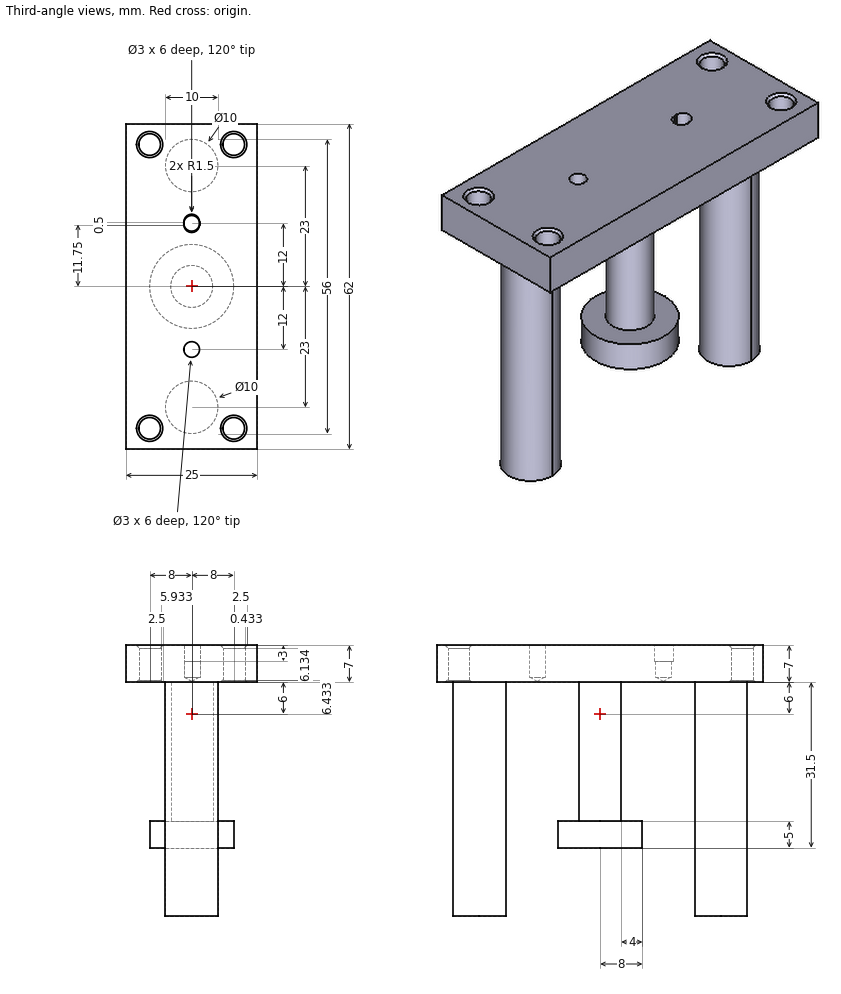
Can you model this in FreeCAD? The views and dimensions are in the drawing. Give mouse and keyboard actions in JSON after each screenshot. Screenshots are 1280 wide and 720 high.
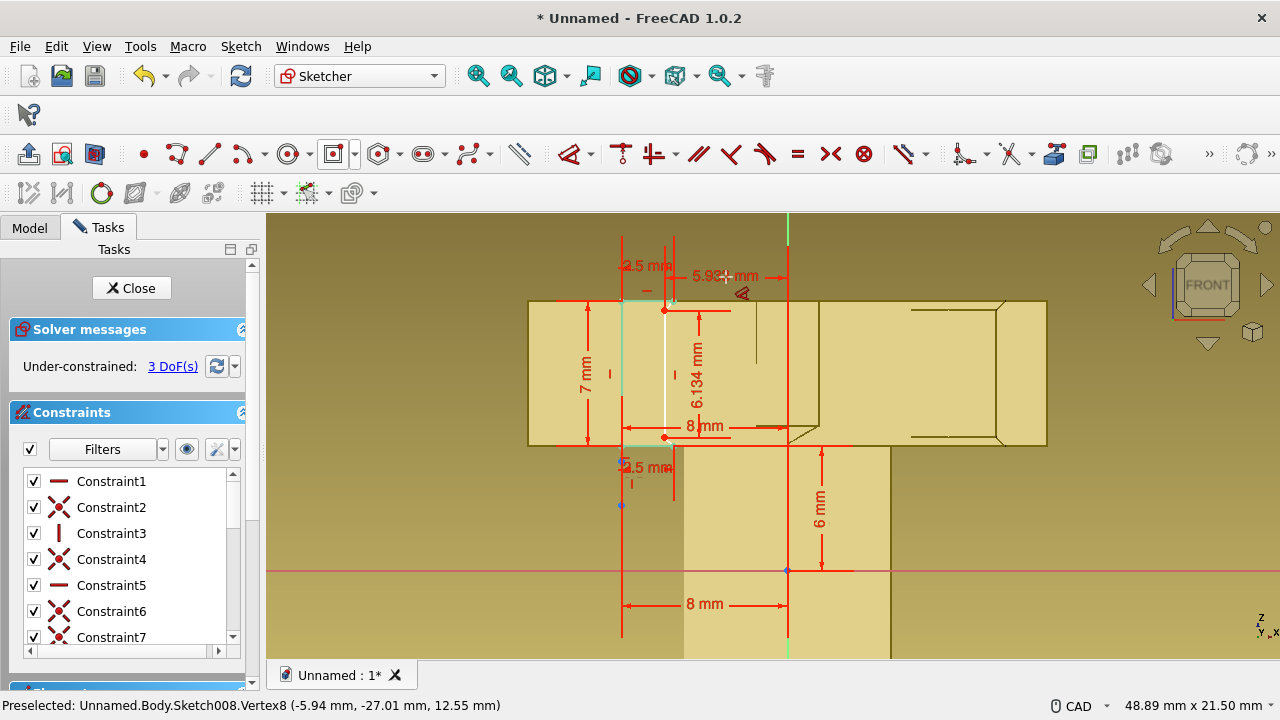
{"action": "left_click", "coordinate": [665, 438]}
{"action": "left_click", "coordinate": [822, 474]}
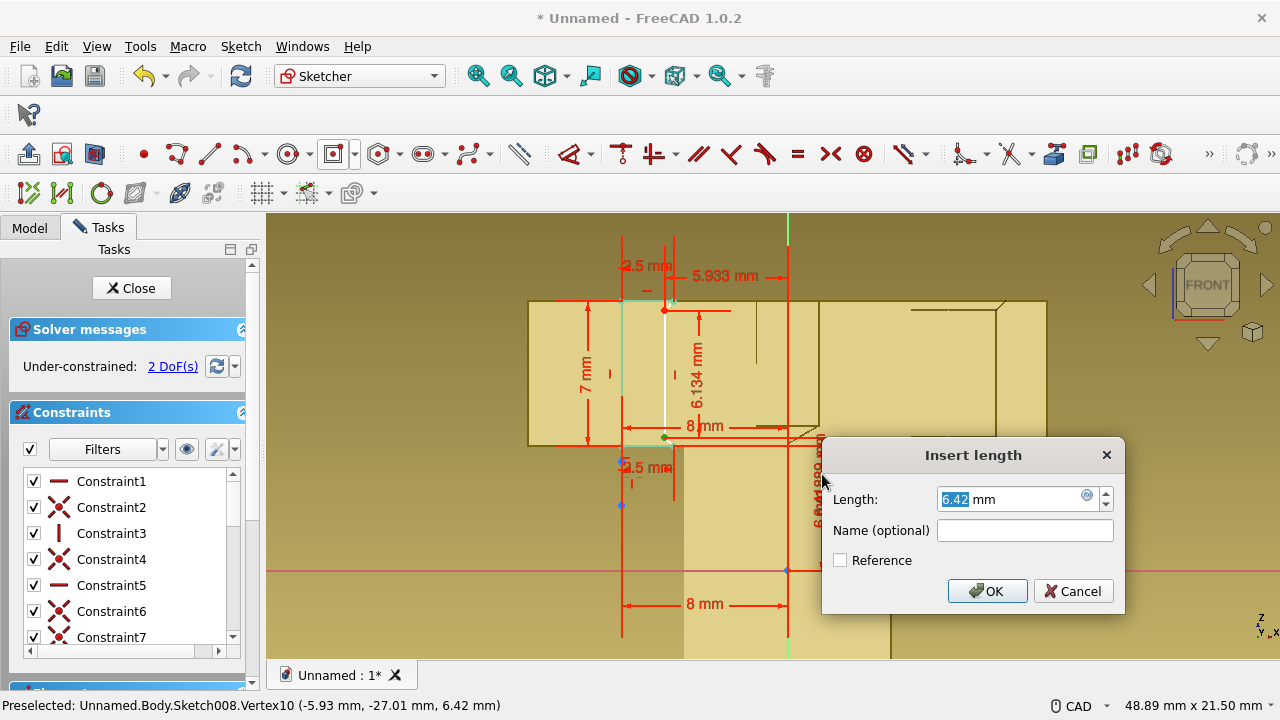
{"action": "type", "text": "6.433"}
{"action": "key", "text": "Return"}
{"action": "key", "text": "Escape"}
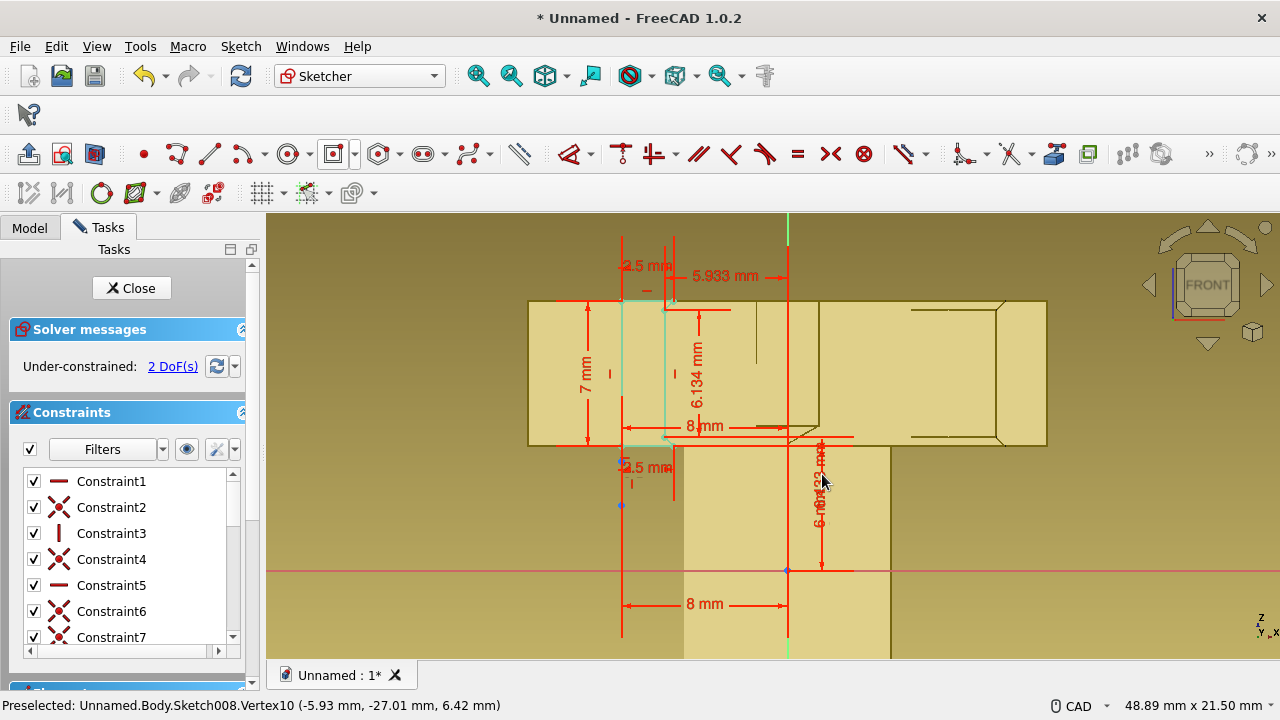
{"action": "left_click", "coordinate": [132, 288]}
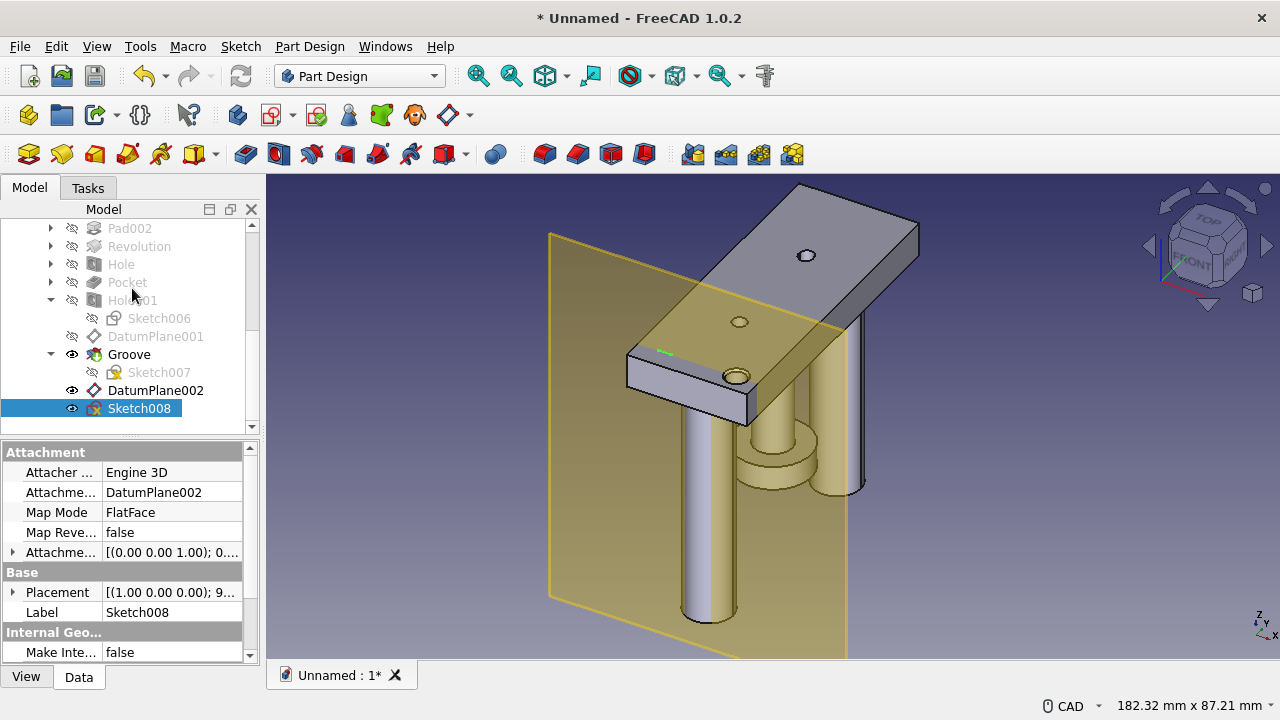
{"action": "left_click", "coordinate": [312, 154]}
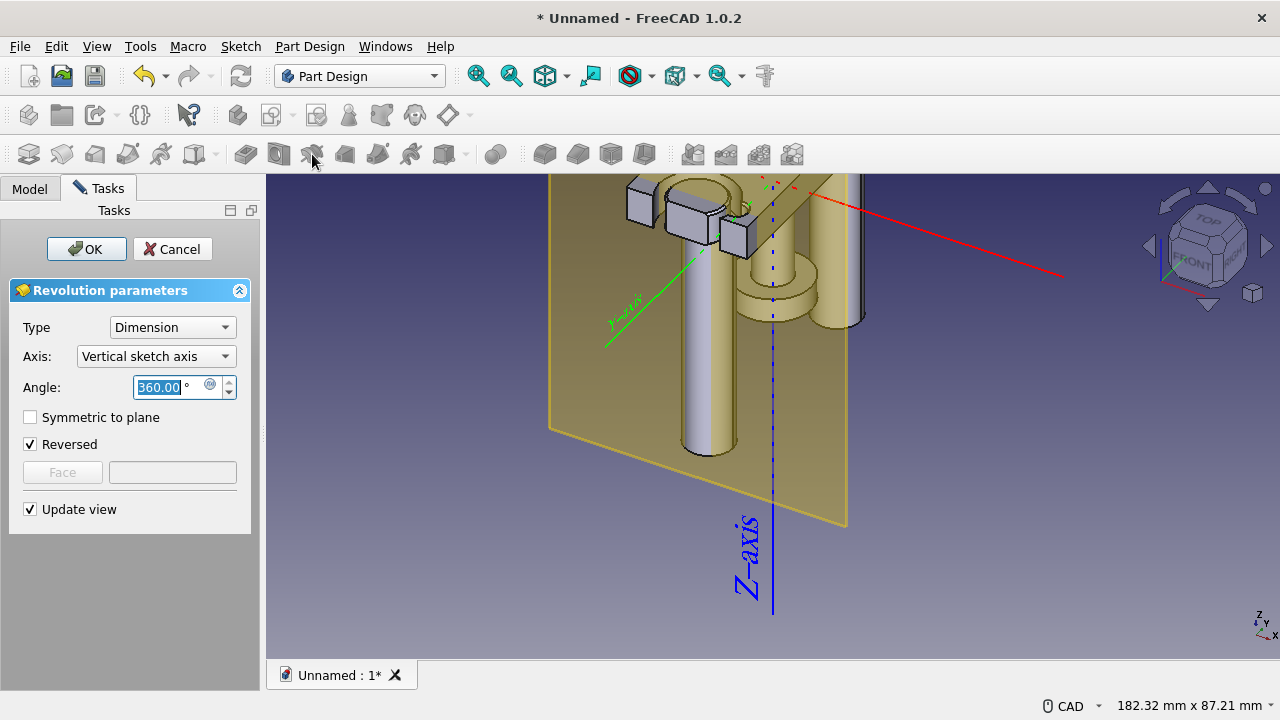
{"action": "left_click", "coordinate": [157, 356]}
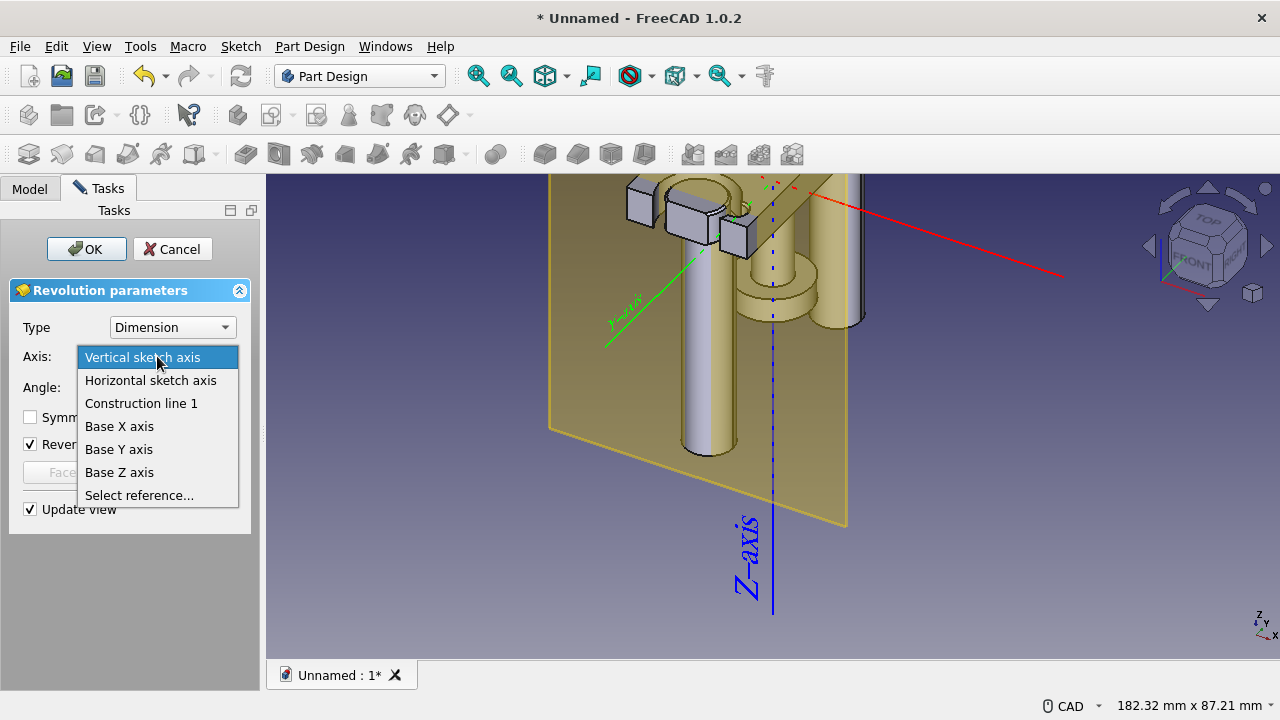
{"action": "left_click", "coordinate": [156, 404]}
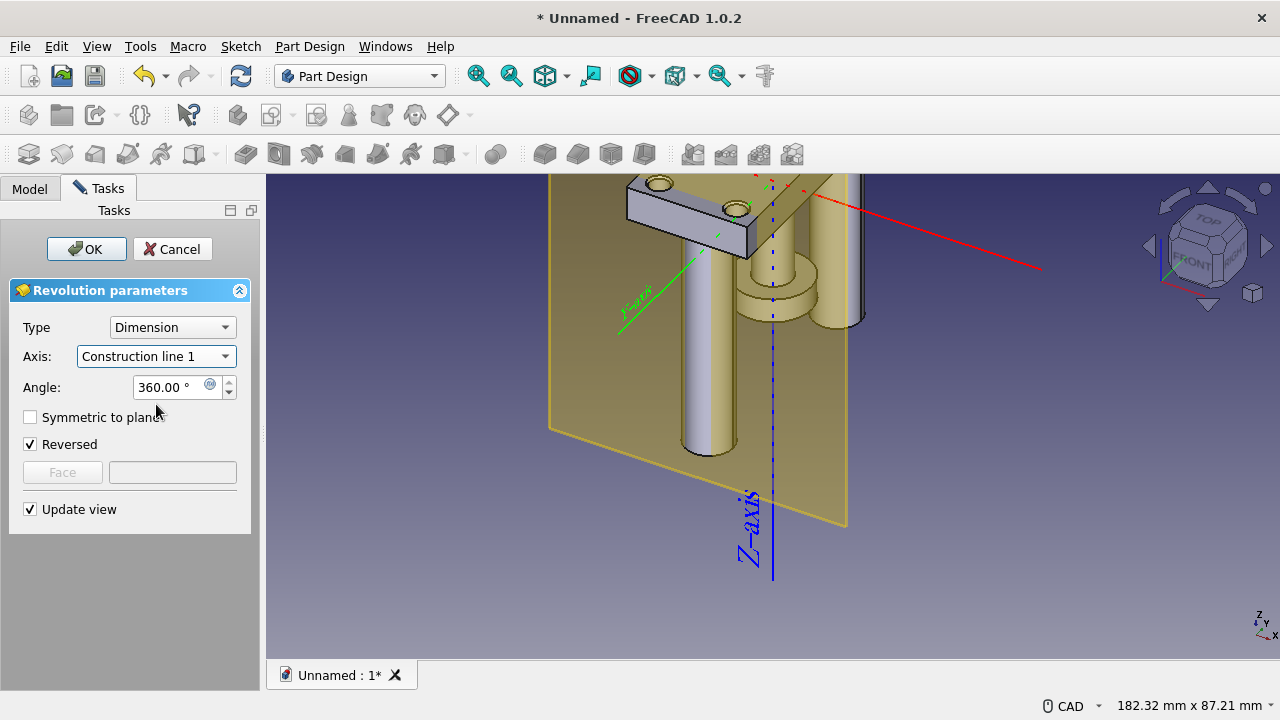
{"action": "left_click", "coordinate": [87, 249]}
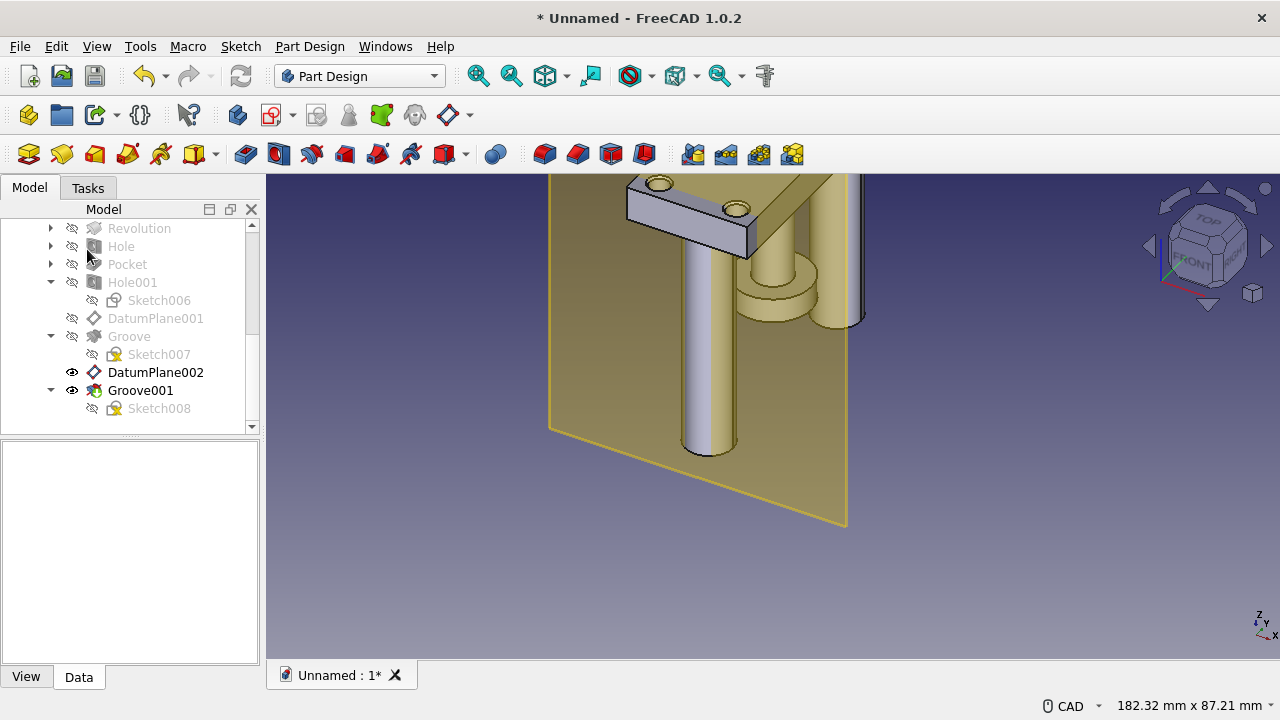
{"action": "left_click", "coordinate": [117, 372]}
{"action": "key", "text": "space"}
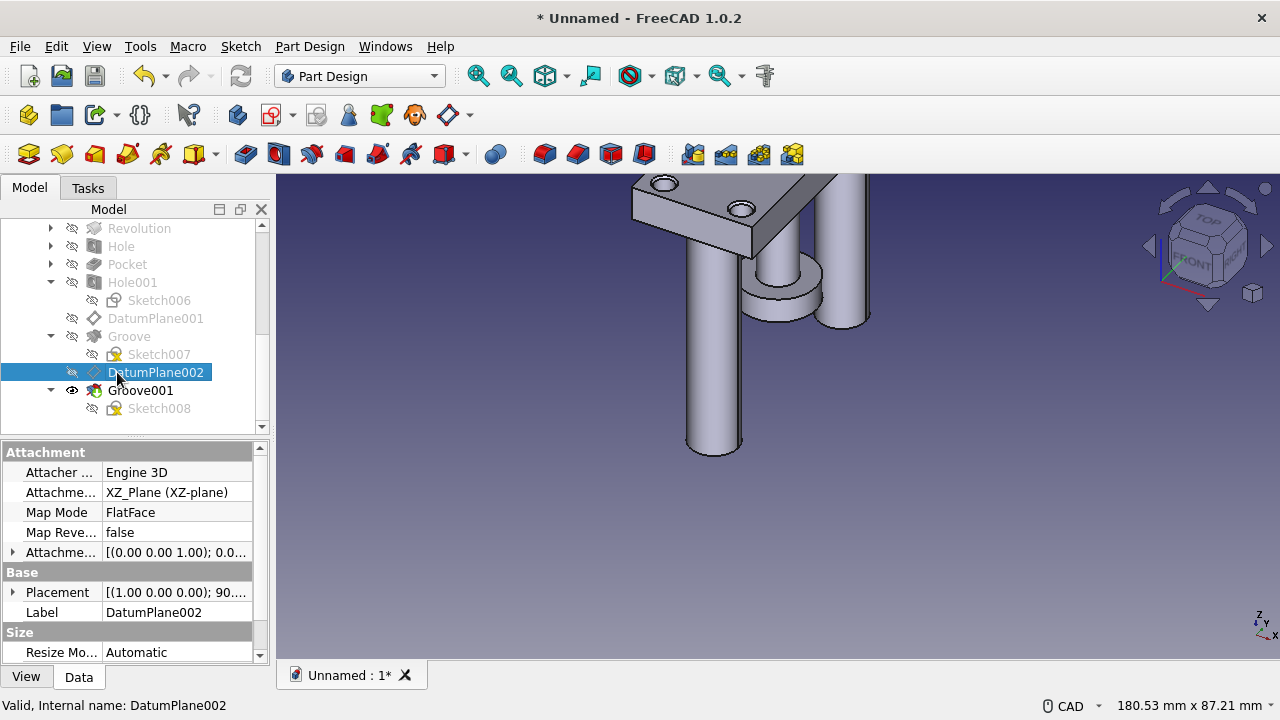
{"action": "left_click", "coordinate": [479, 76]}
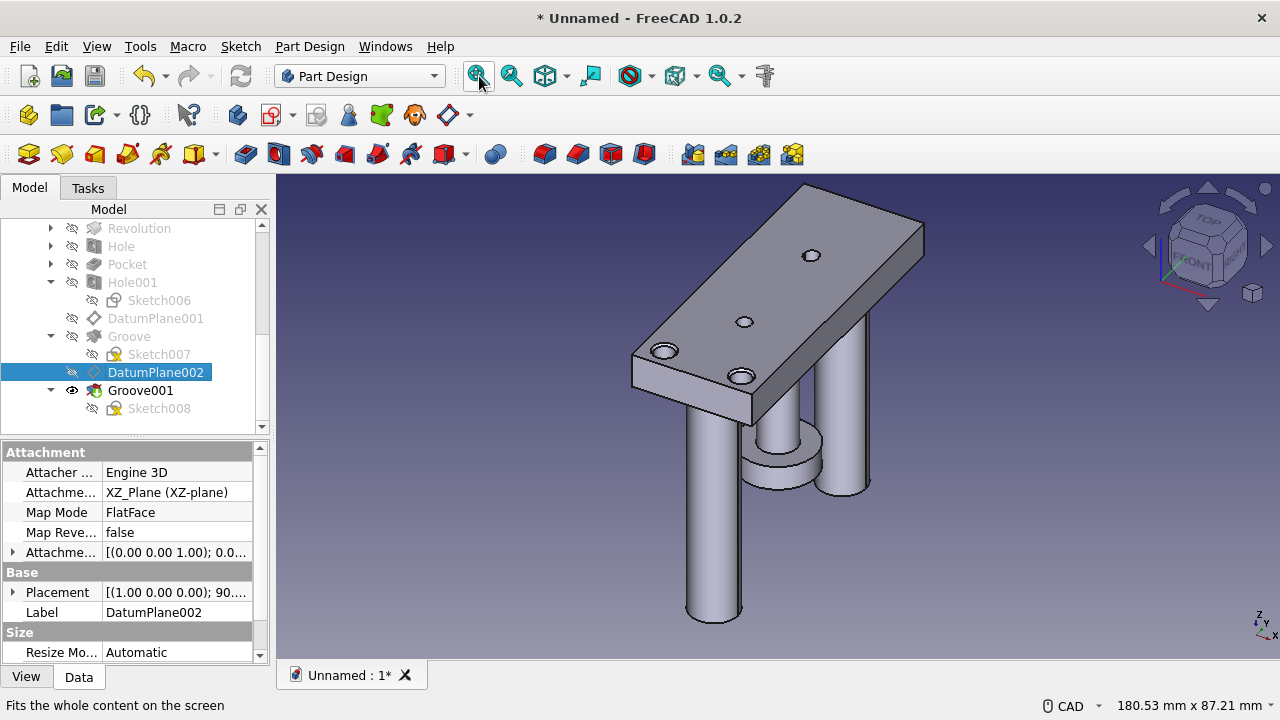
{"action": "scroll", "coordinate": [141, 314], "scroll_direction": "down", "scroll_amount": 3}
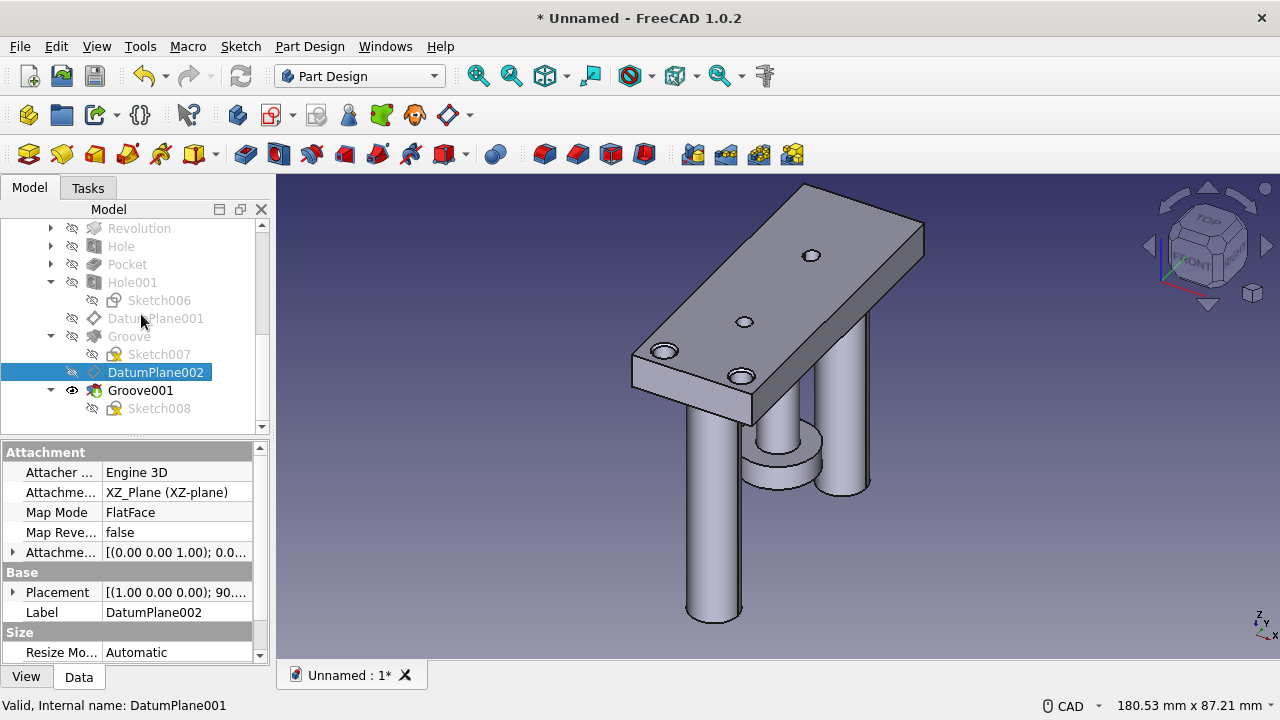
{"action": "scroll", "coordinate": [141, 314], "scroll_direction": "up", "scroll_amount": 15}